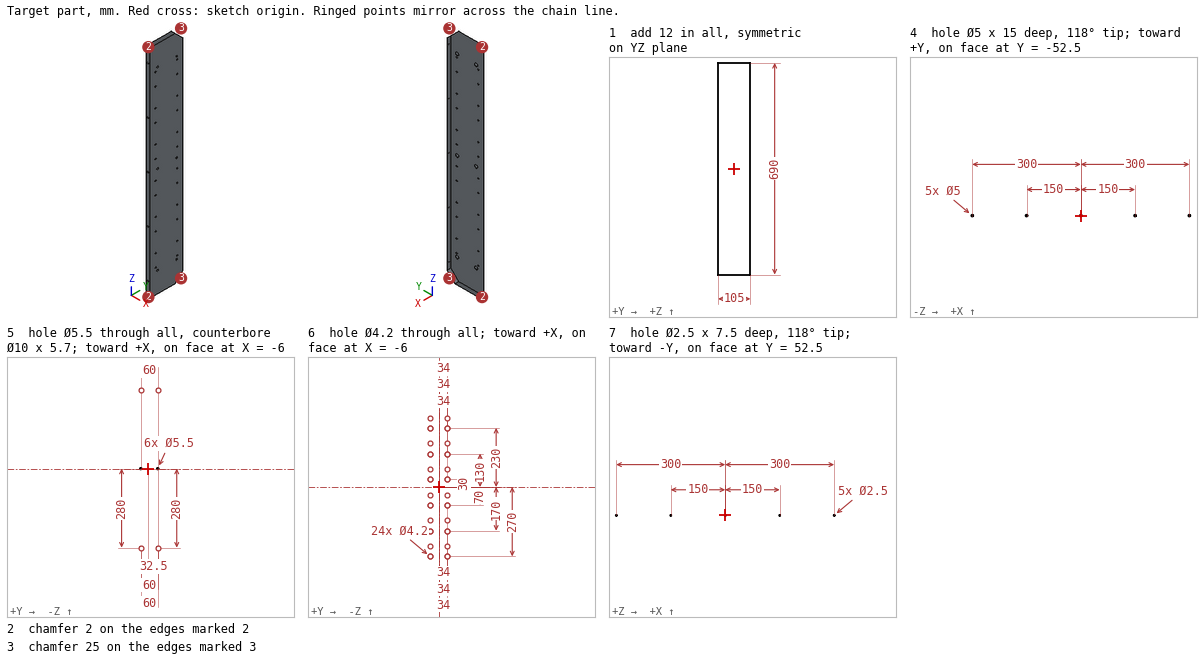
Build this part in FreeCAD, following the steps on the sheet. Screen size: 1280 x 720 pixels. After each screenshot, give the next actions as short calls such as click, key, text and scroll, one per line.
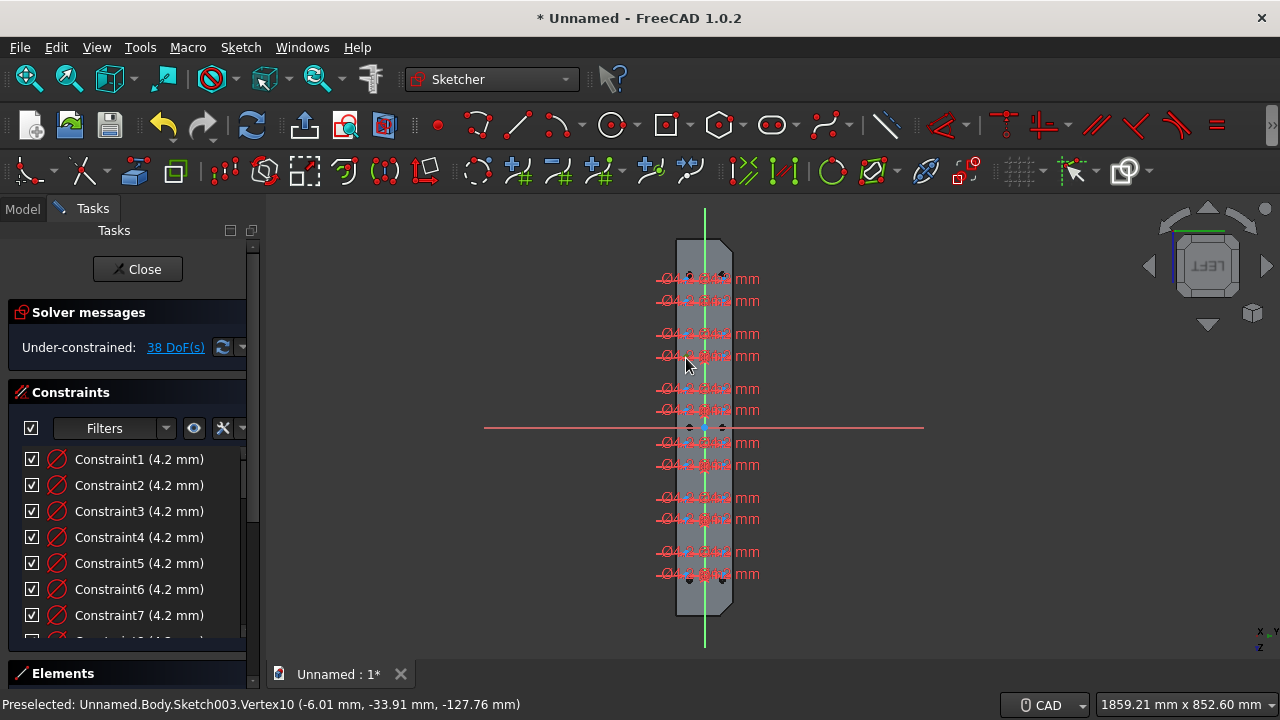
click(686, 500)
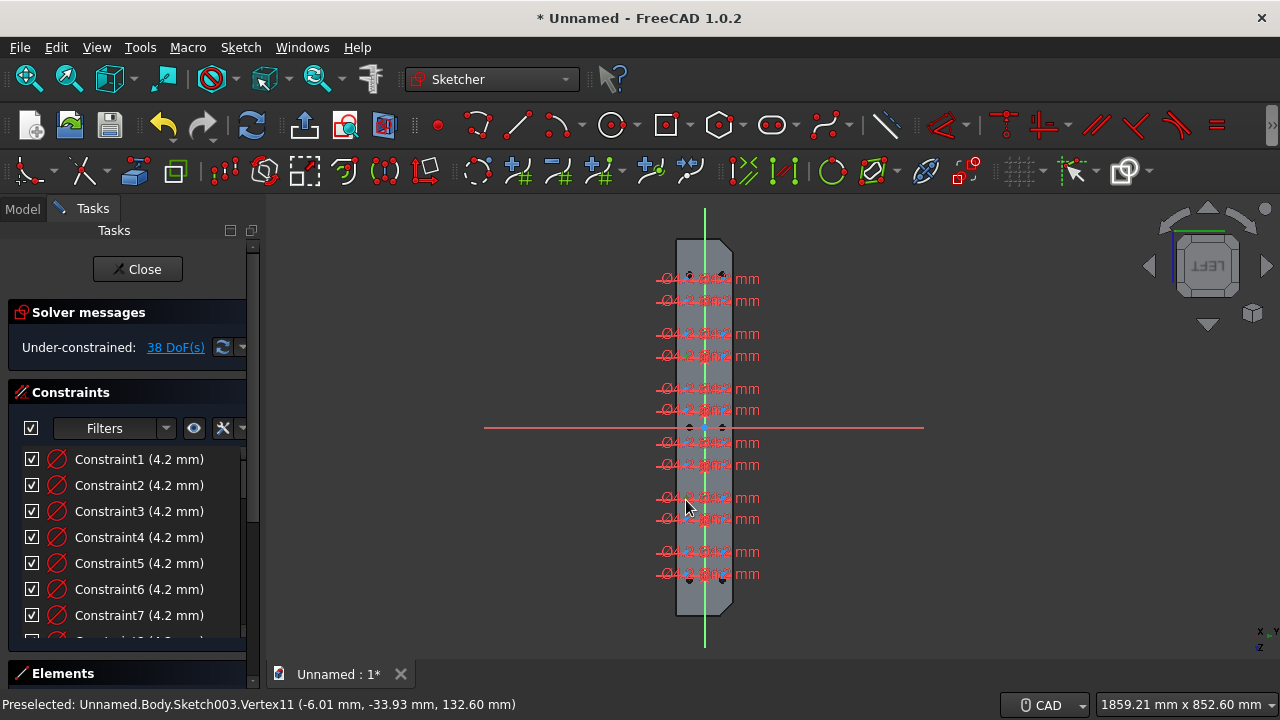
click(529, 428)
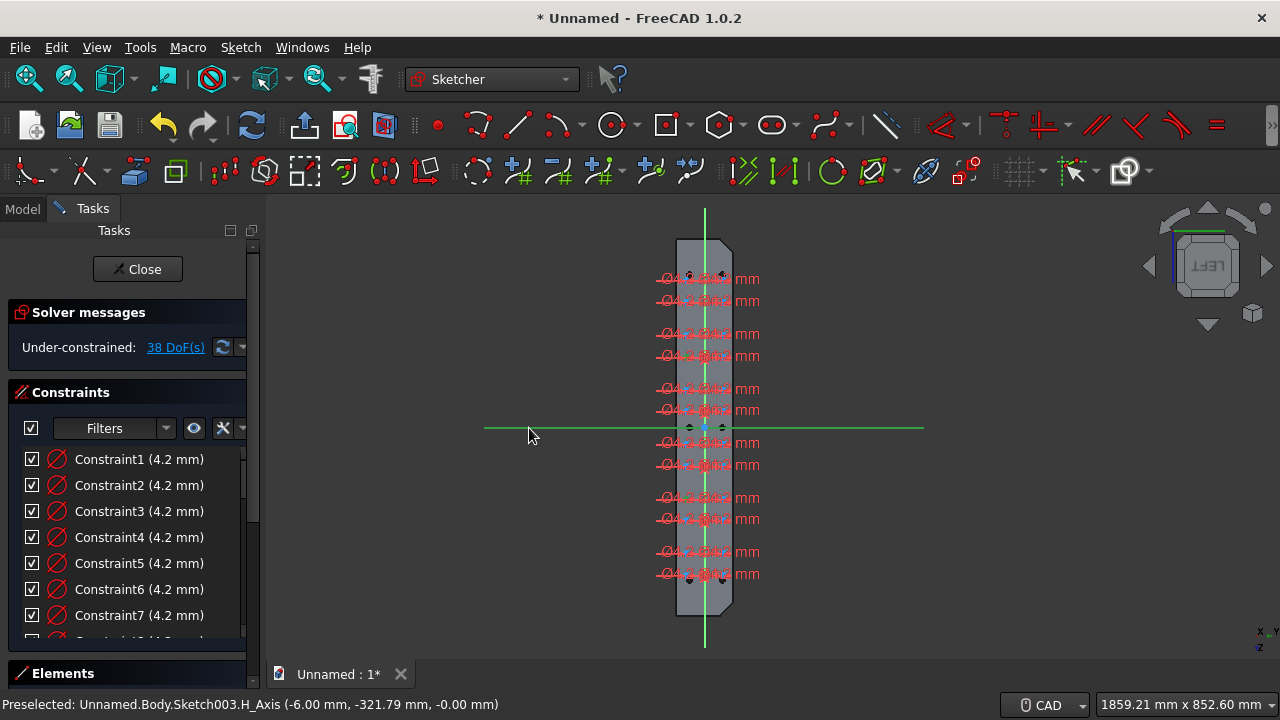
key(s)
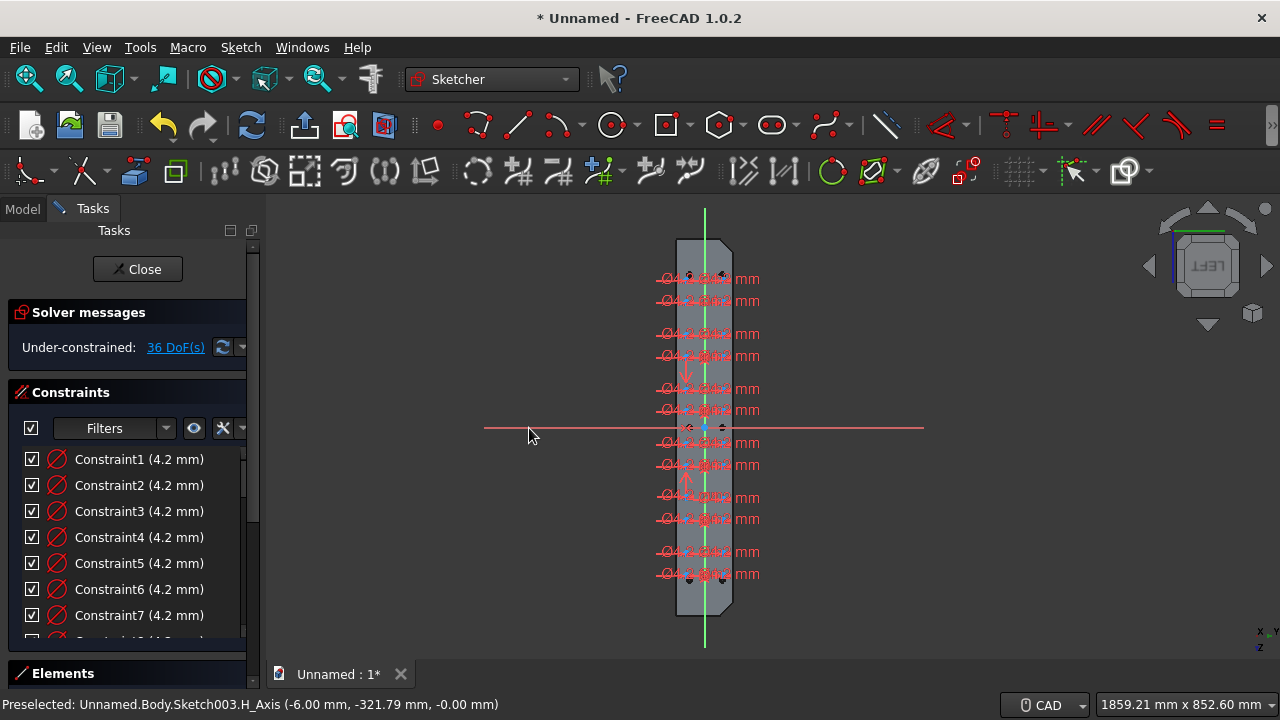
click(723, 358)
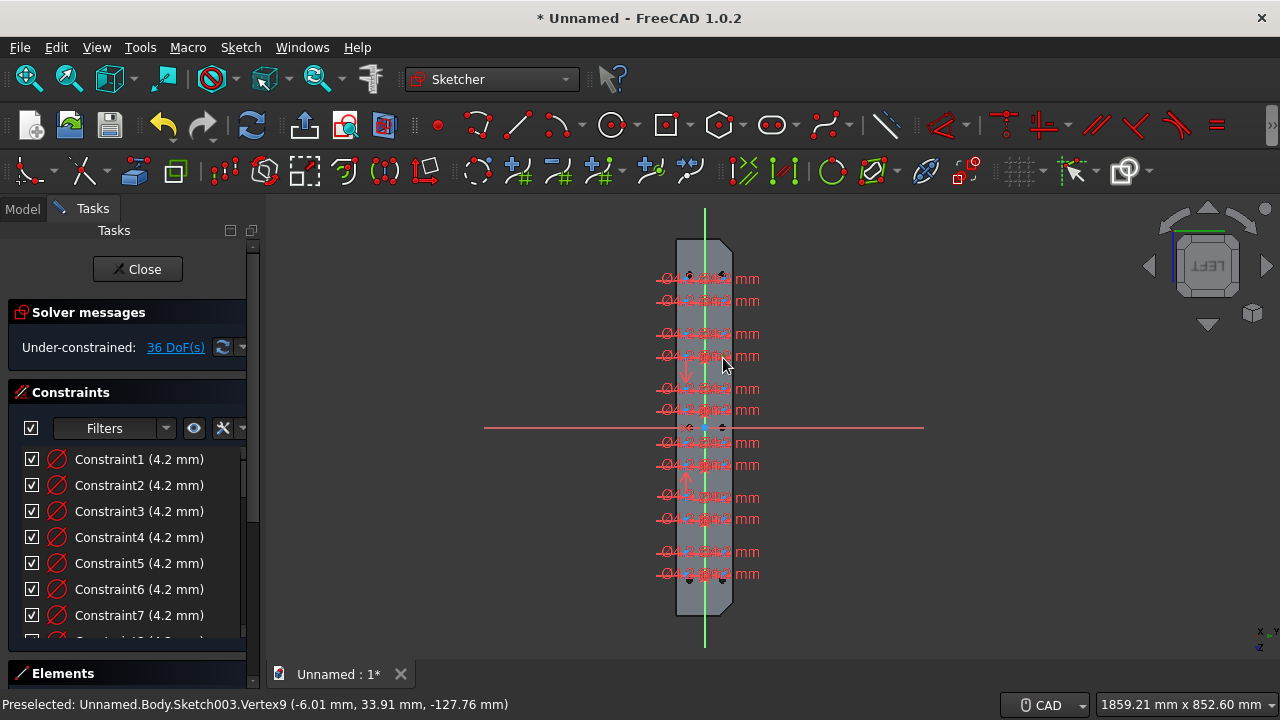
click(723, 500)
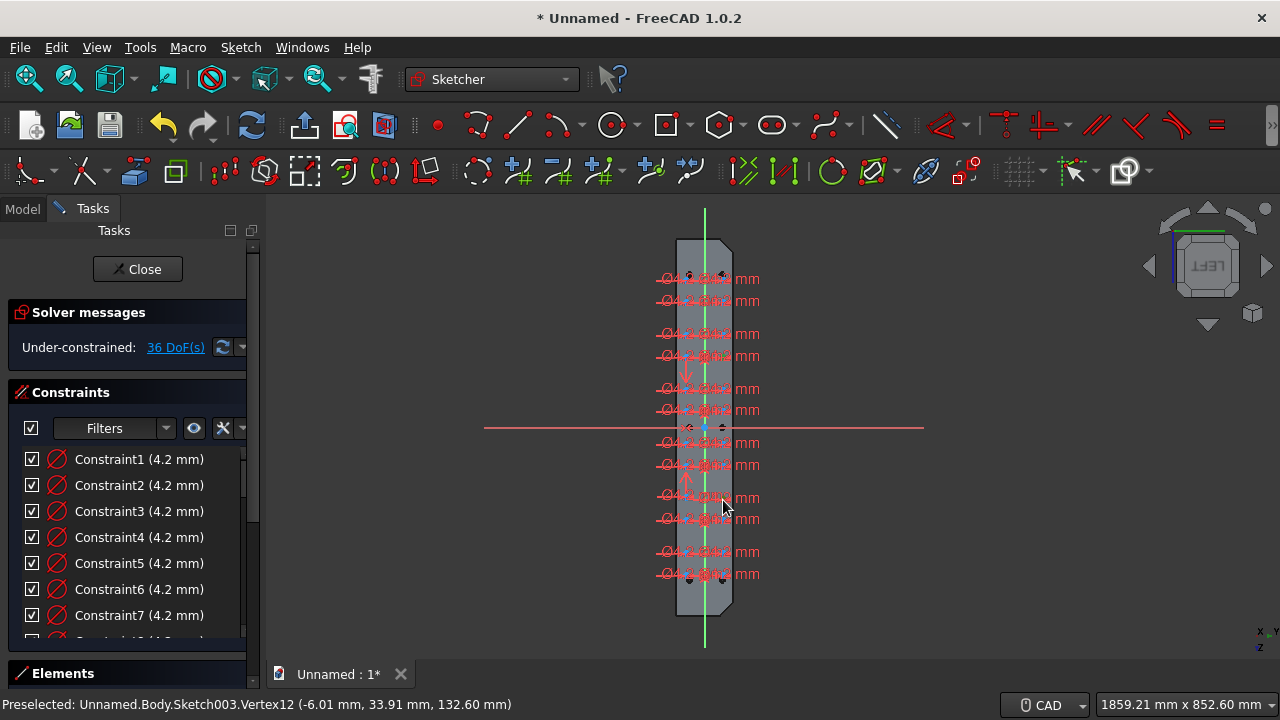
click(529, 428)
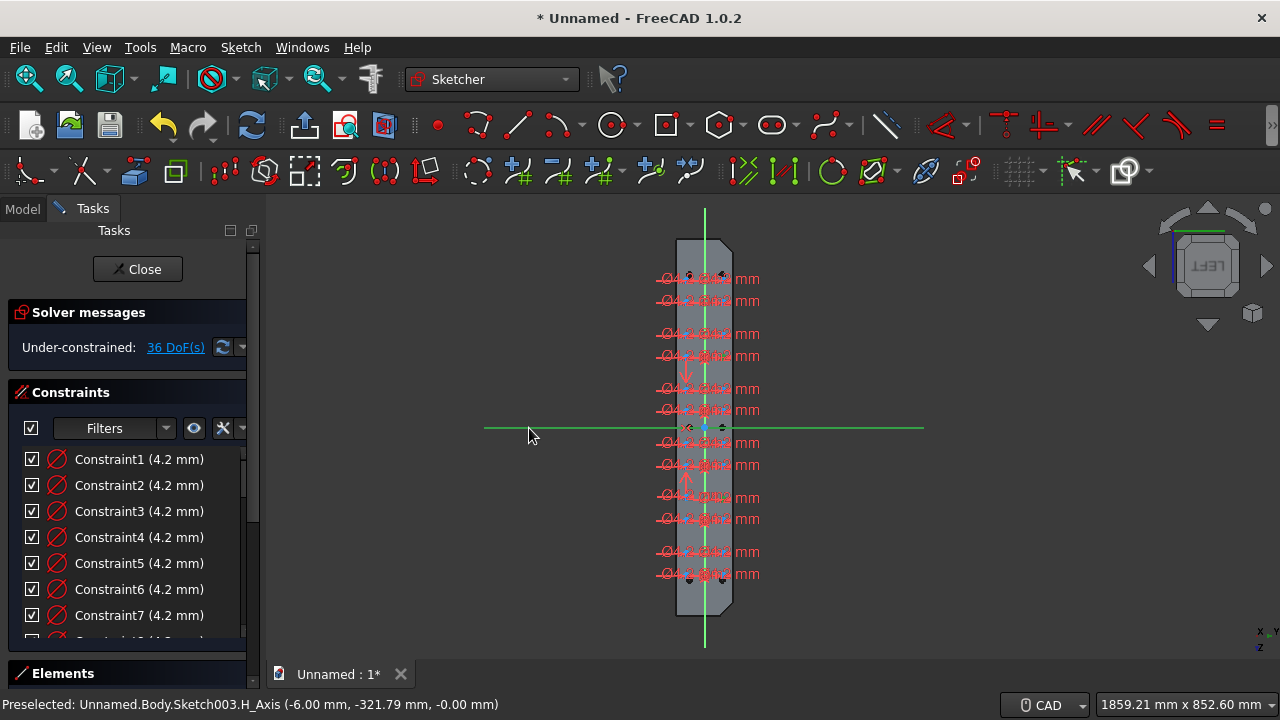
key(s)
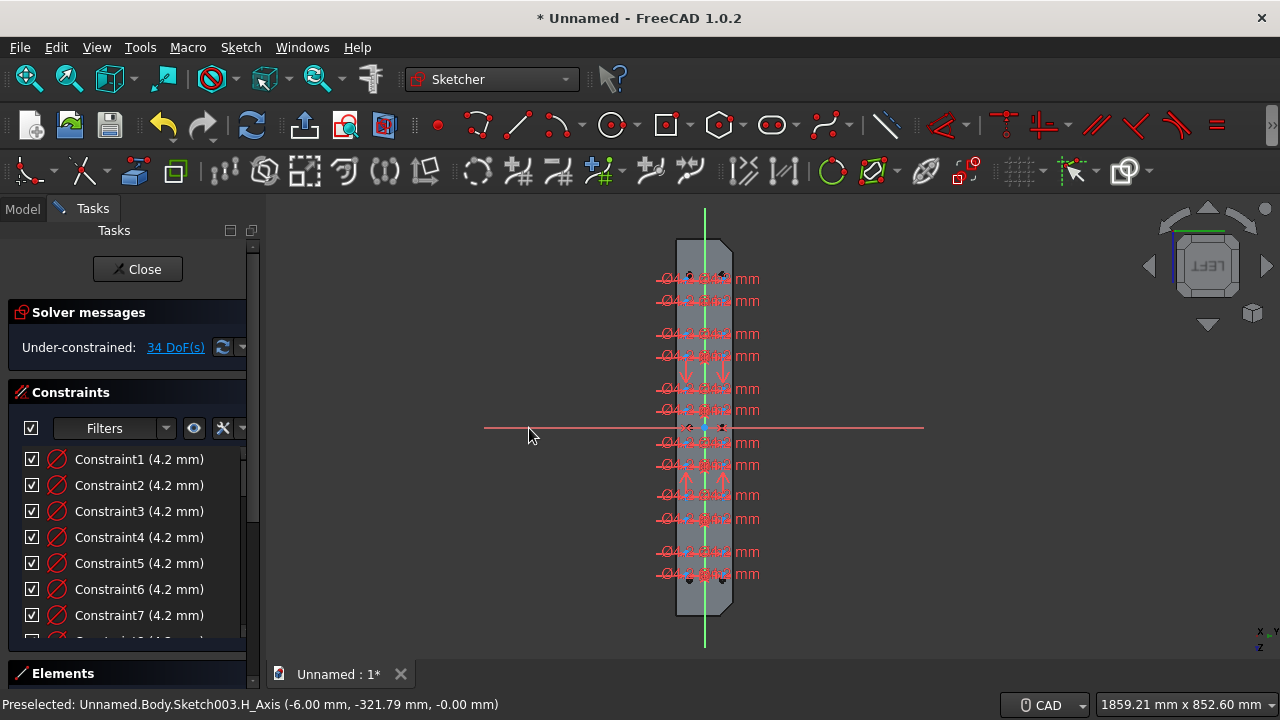
click(686, 412)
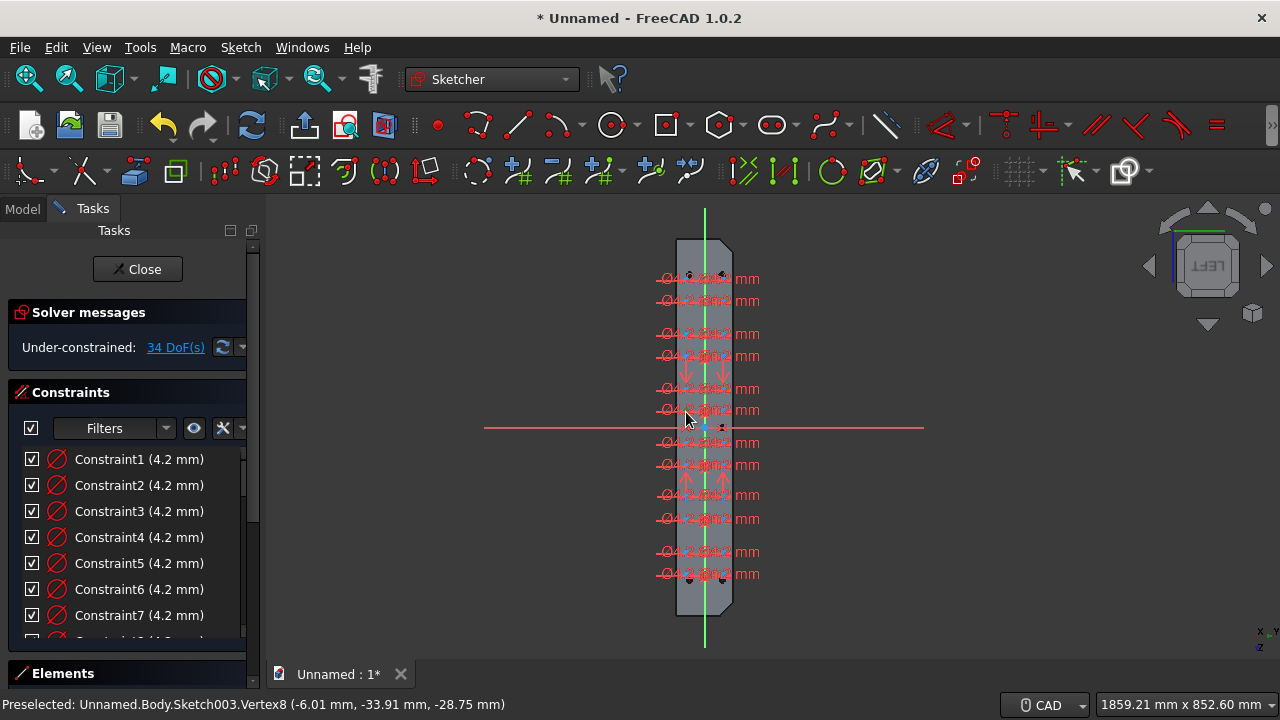
click(686, 445)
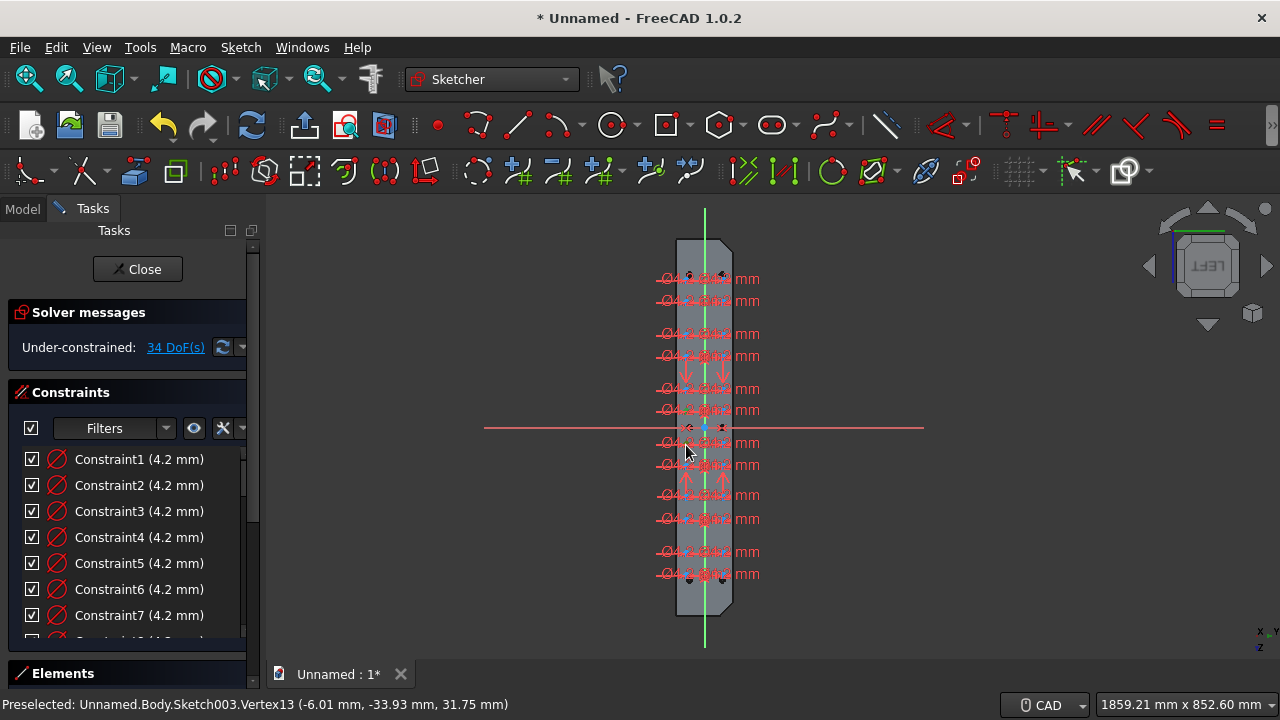
click(529, 428)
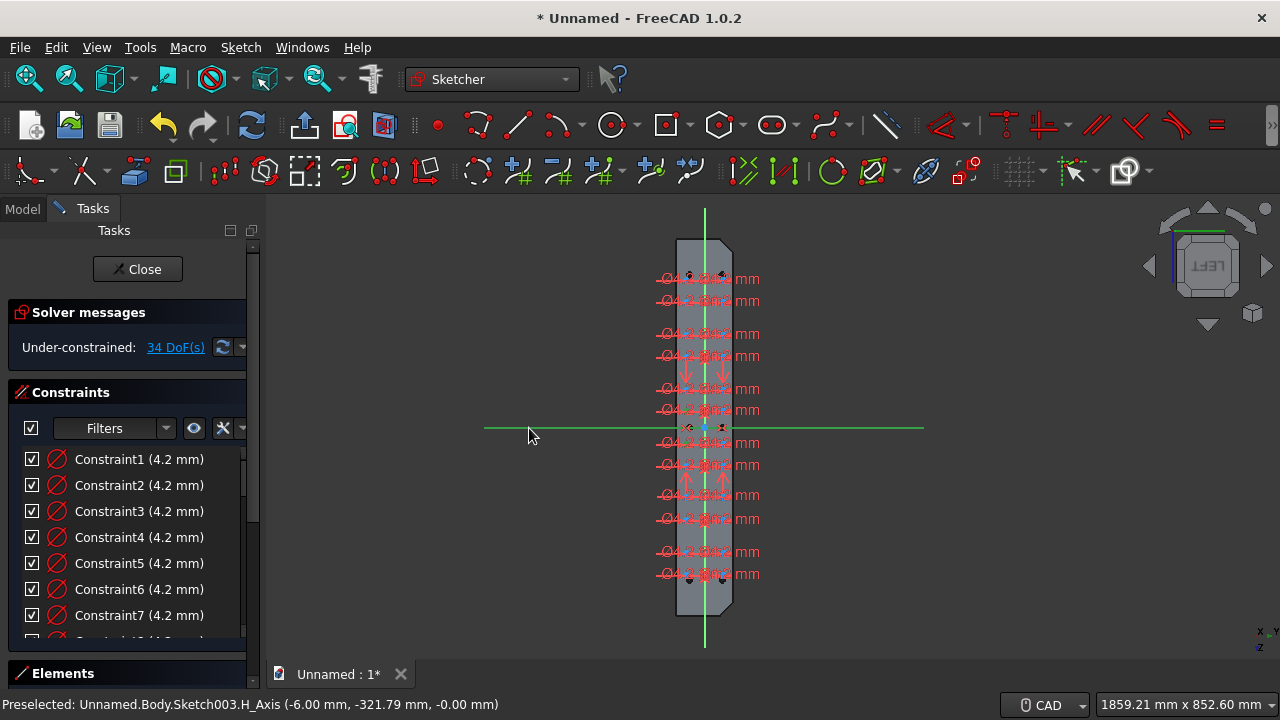
key(s)